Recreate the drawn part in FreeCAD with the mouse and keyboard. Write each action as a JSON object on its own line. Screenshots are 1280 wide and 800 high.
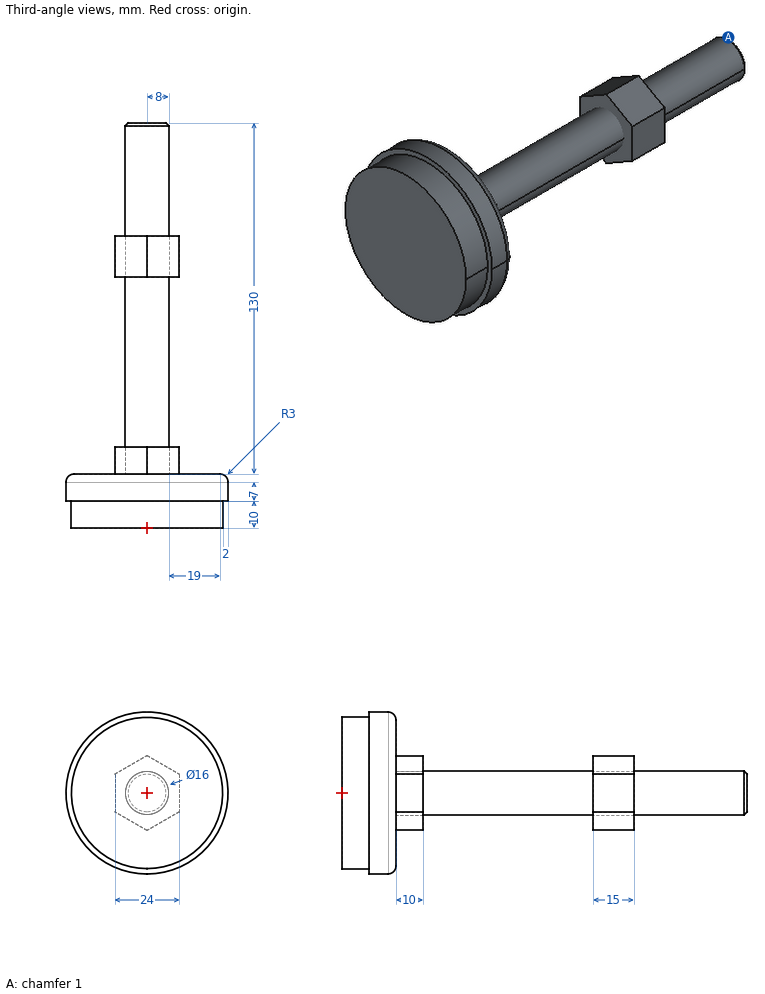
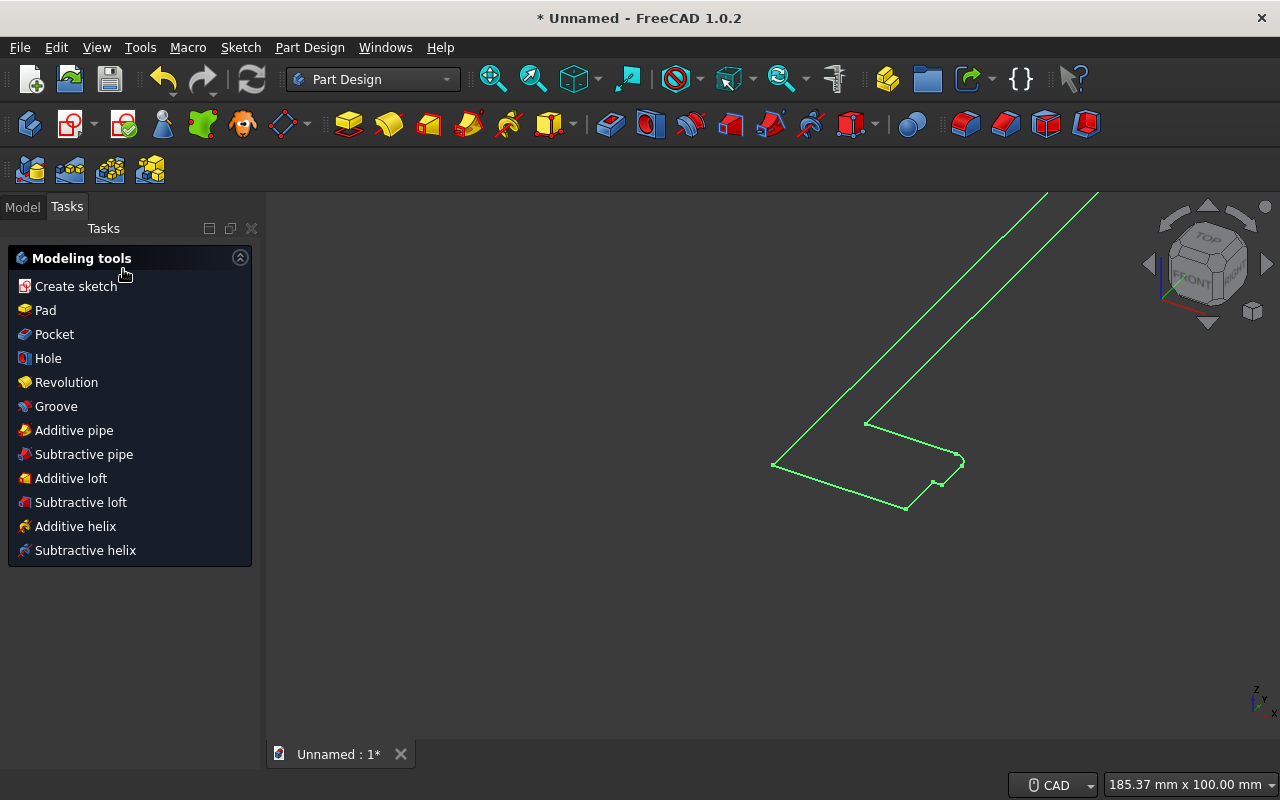
{"action": "left_click", "coordinate": [390, 124]}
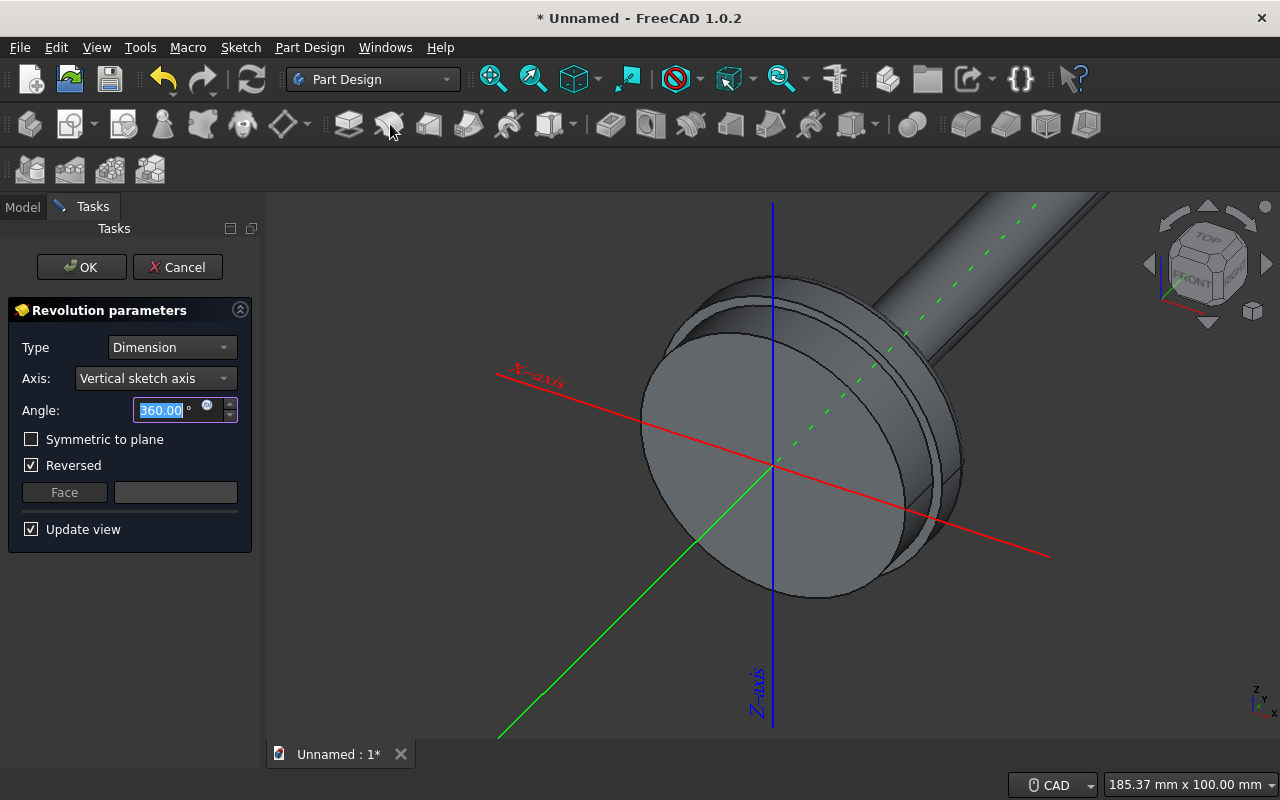
{"action": "left_click", "coordinate": [82, 267]}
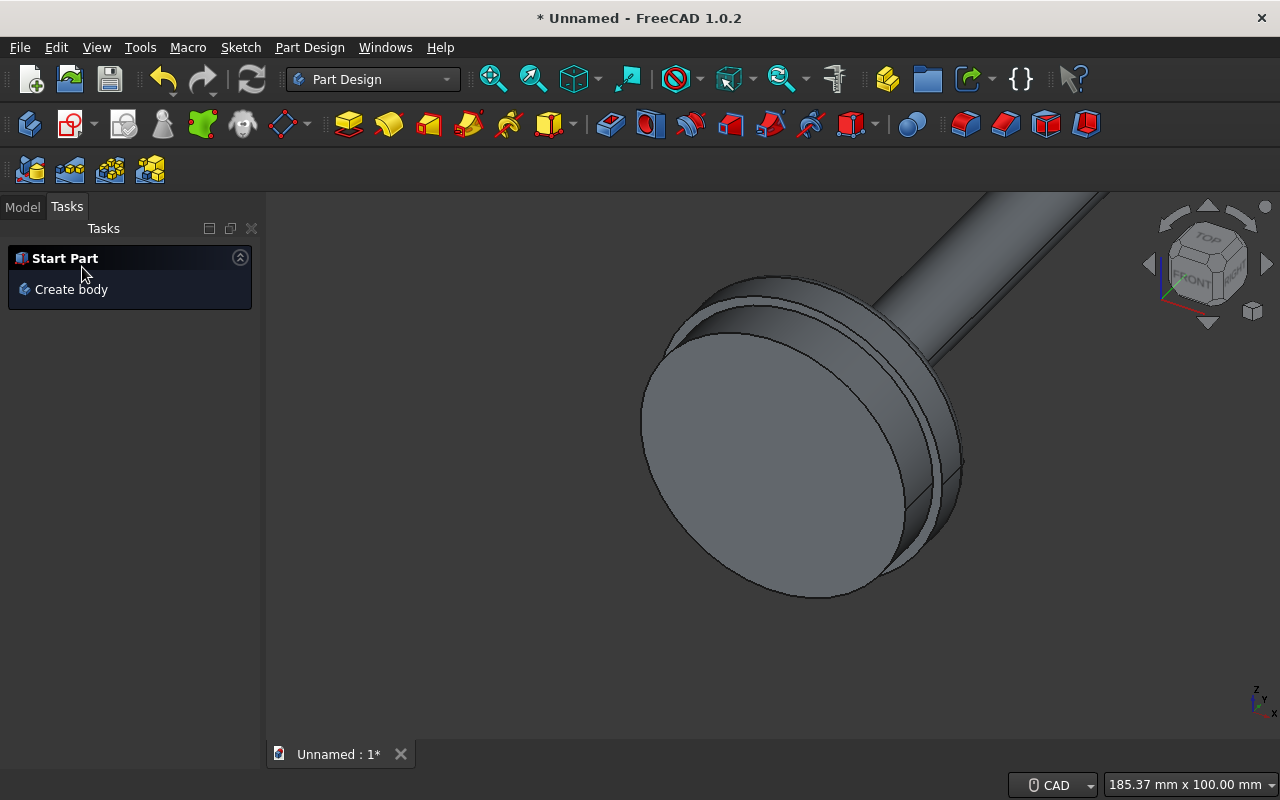
{"action": "left_click", "coordinate": [494, 80]}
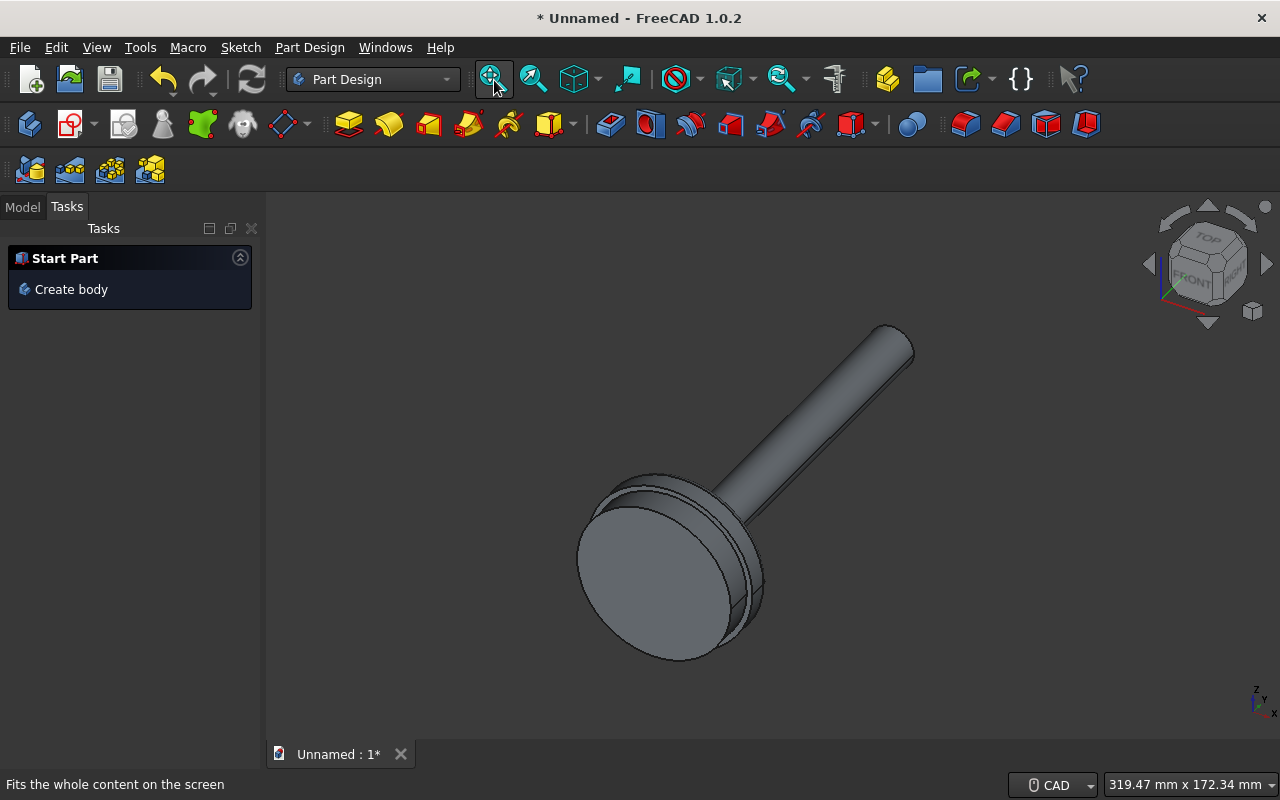
{"action": "key", "text": "0"}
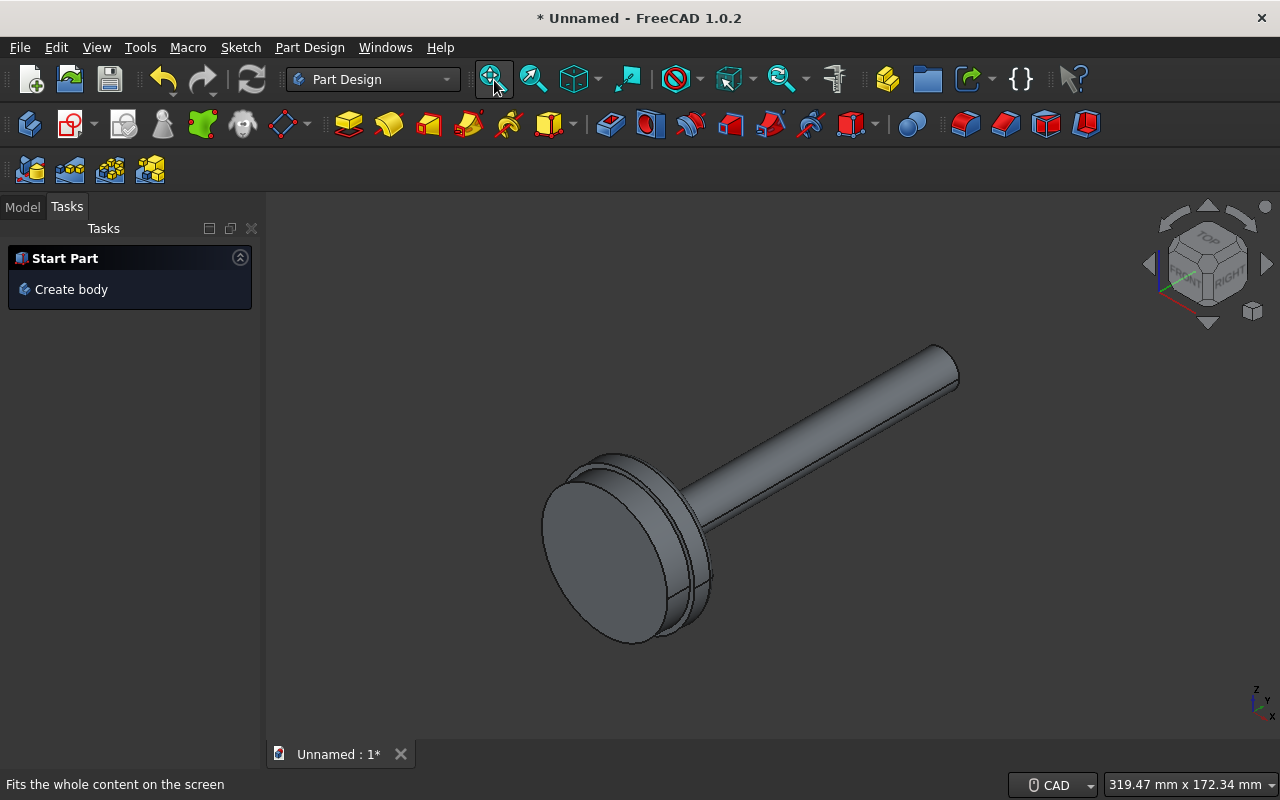
{"action": "left_click", "coordinate": [936, 344]}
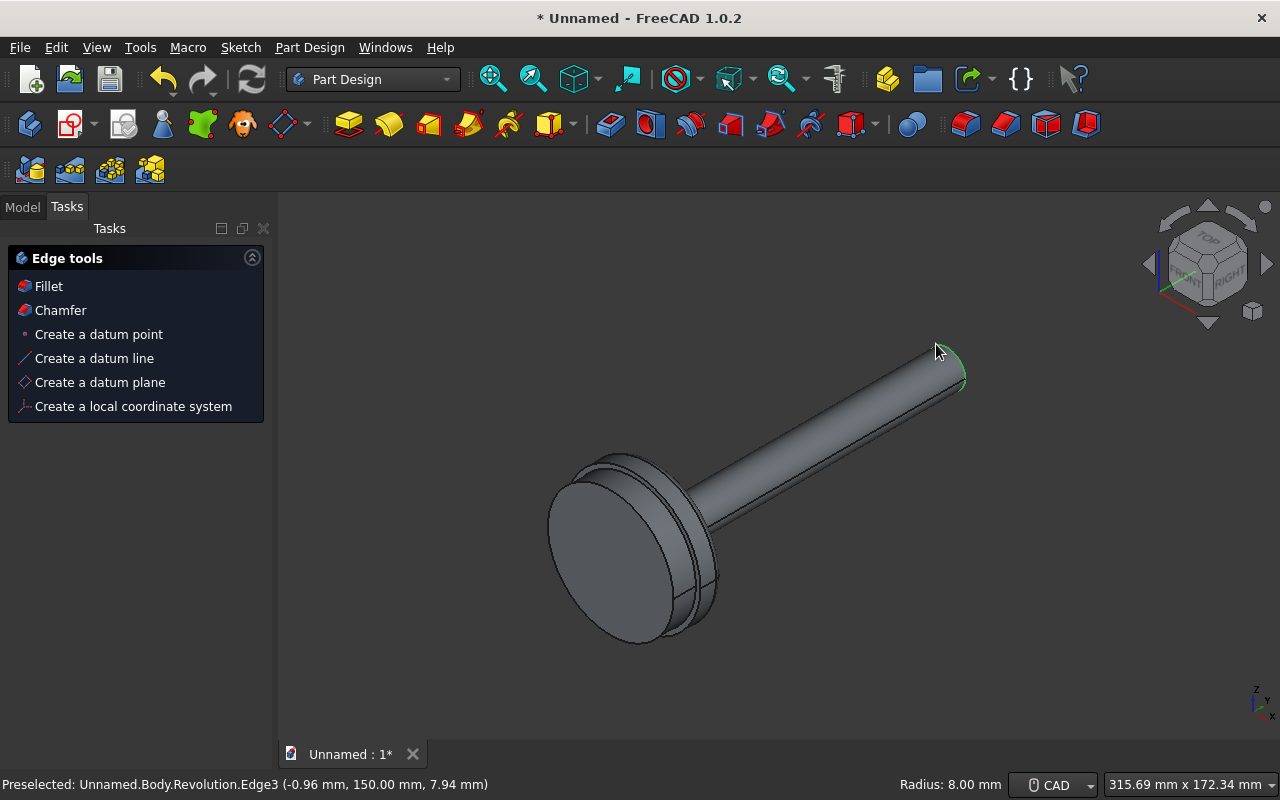
{"action": "left_click", "coordinate": [1006, 124]}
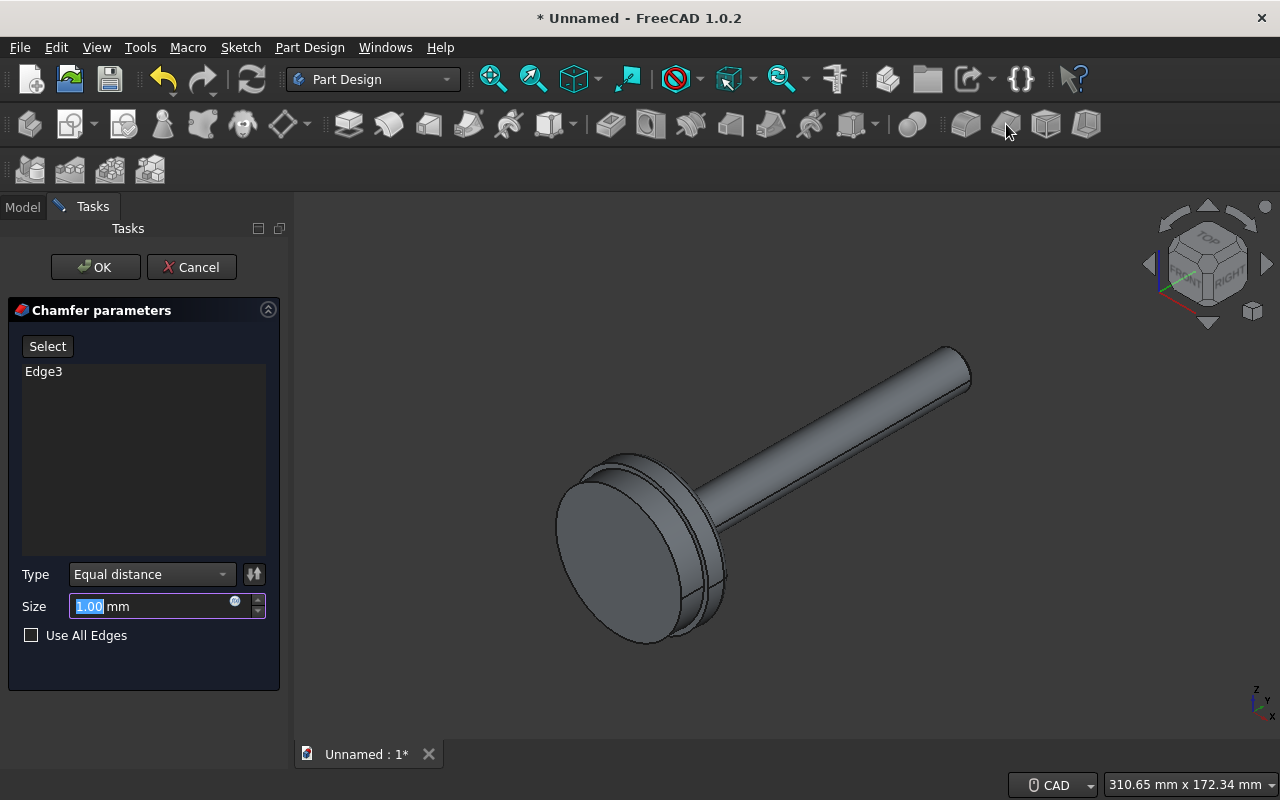
{"action": "type", "text": "1"}
{"action": "key", "text": "Tab"}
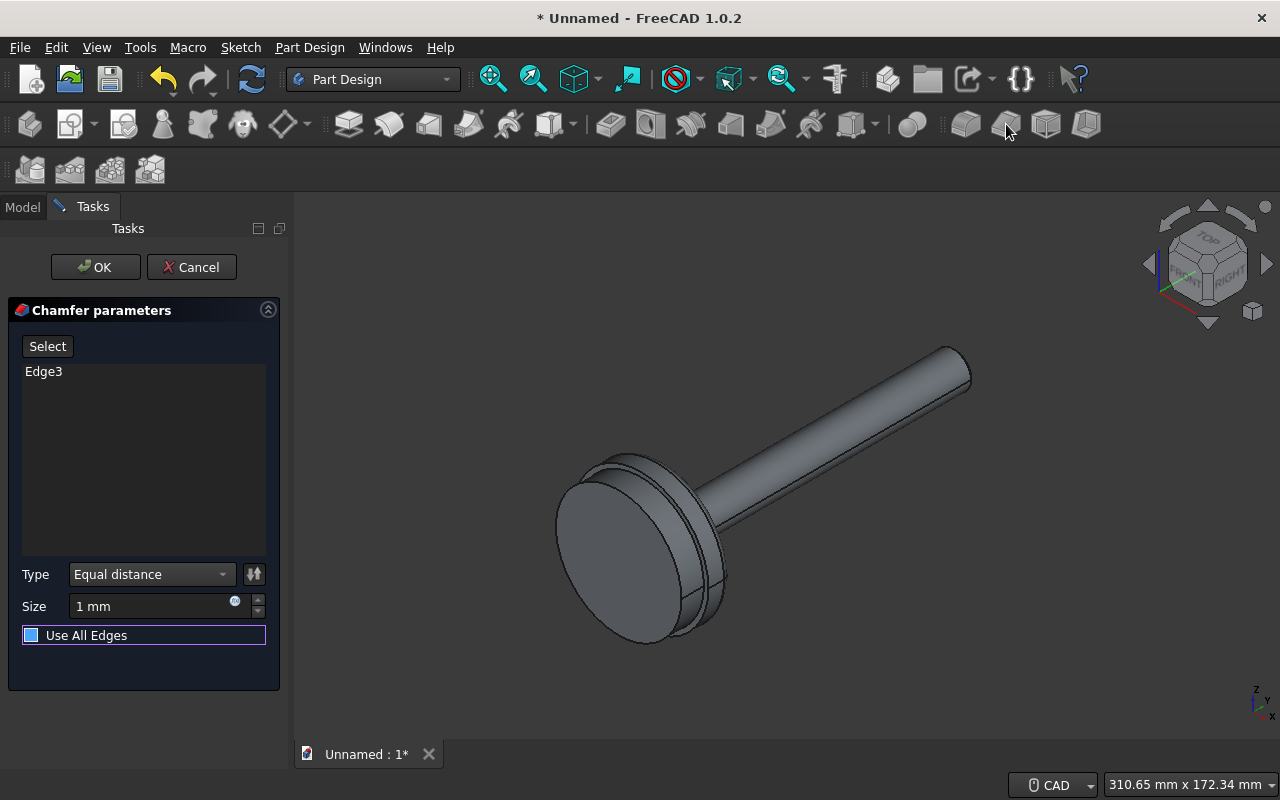
{"action": "left_click", "coordinate": [96, 267]}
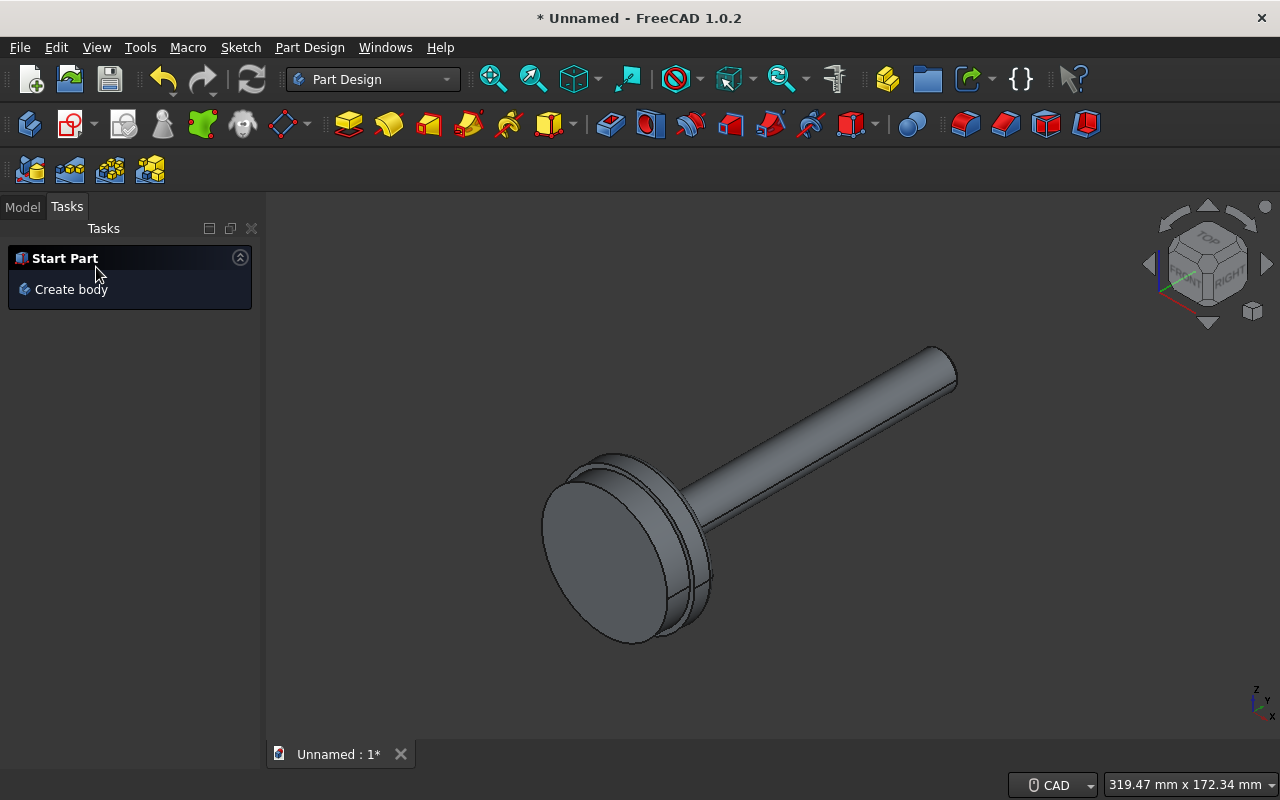
{"action": "left_click", "coordinate": [30, 124]}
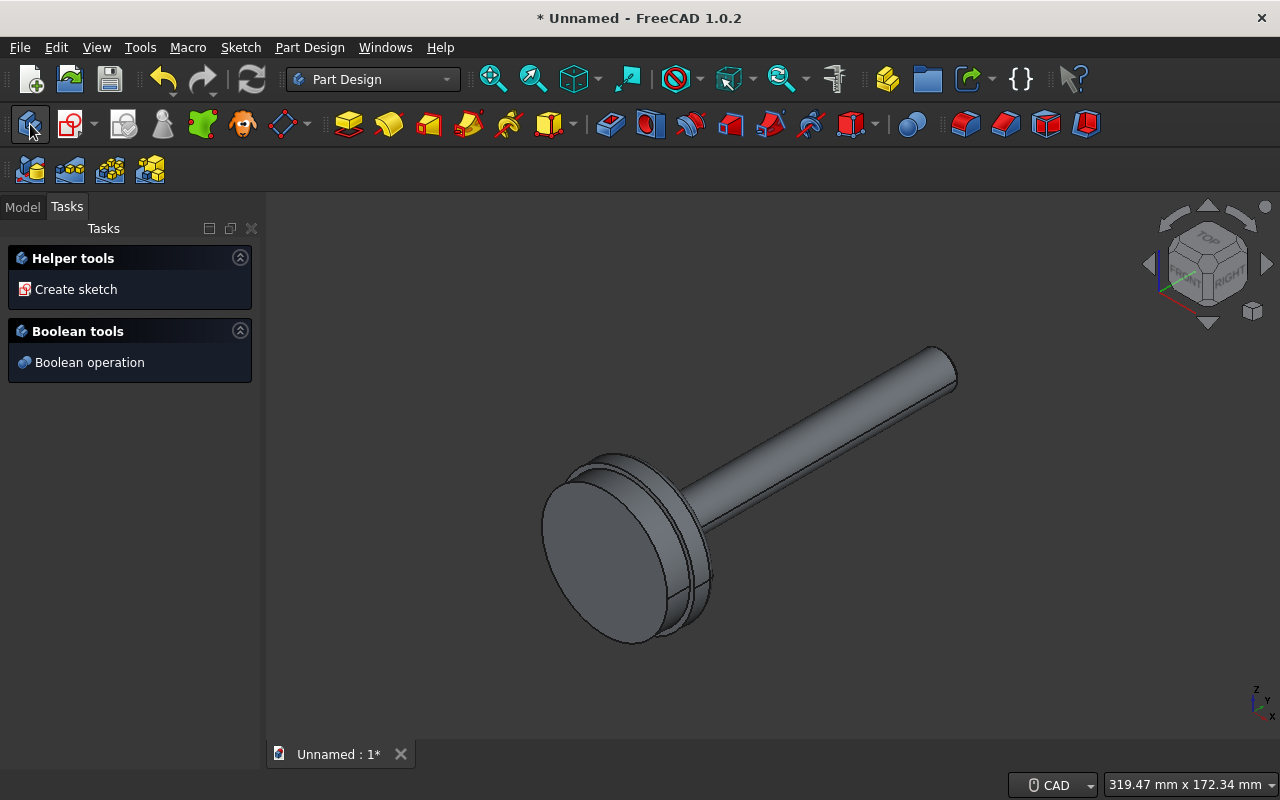
{"action": "left_click", "coordinate": [23, 206]}